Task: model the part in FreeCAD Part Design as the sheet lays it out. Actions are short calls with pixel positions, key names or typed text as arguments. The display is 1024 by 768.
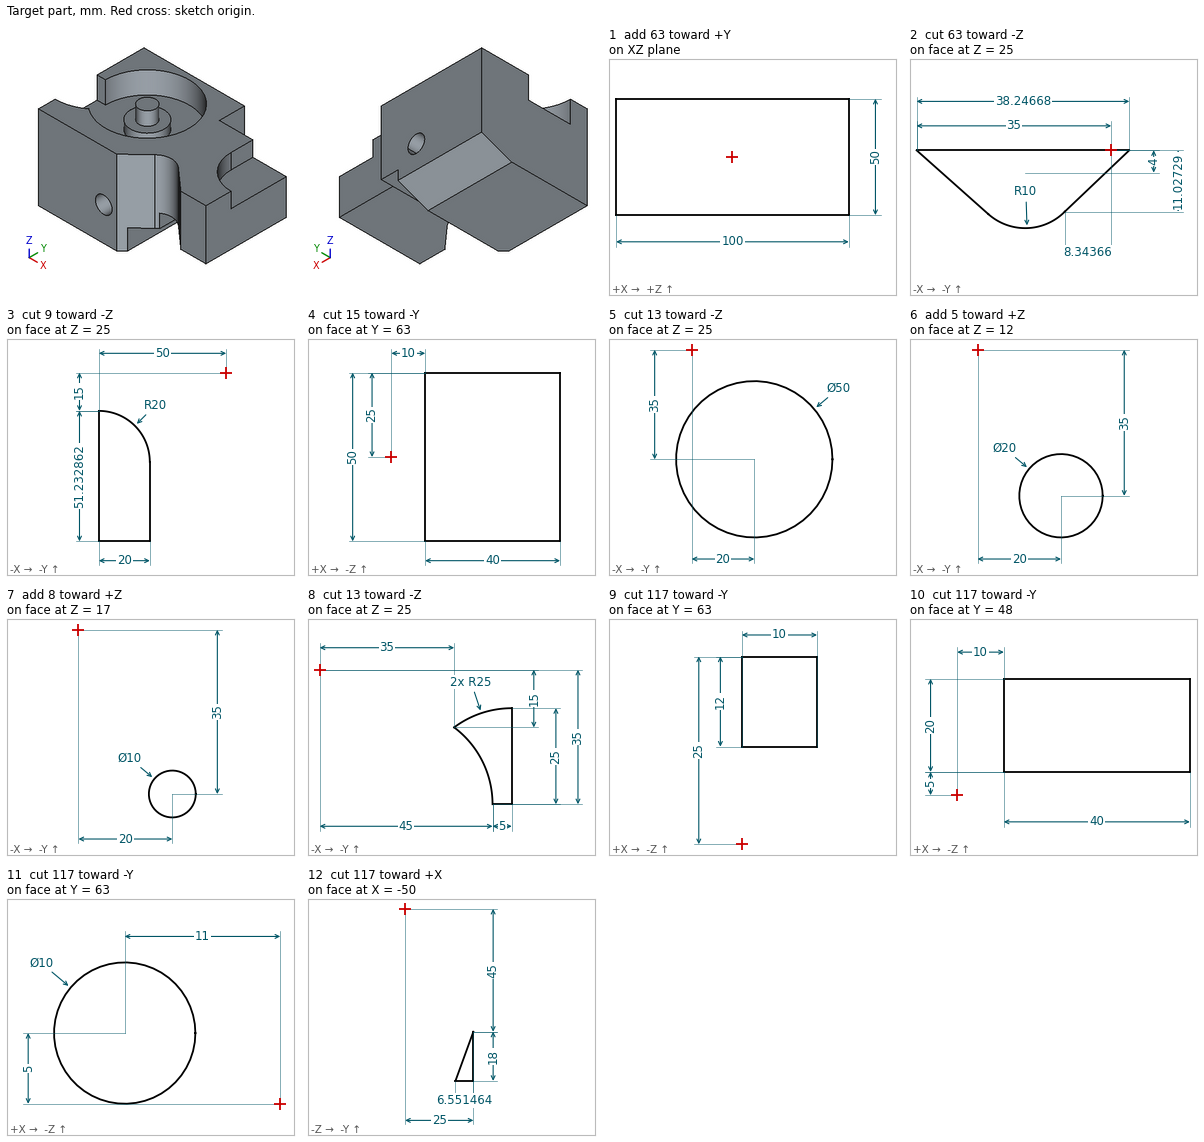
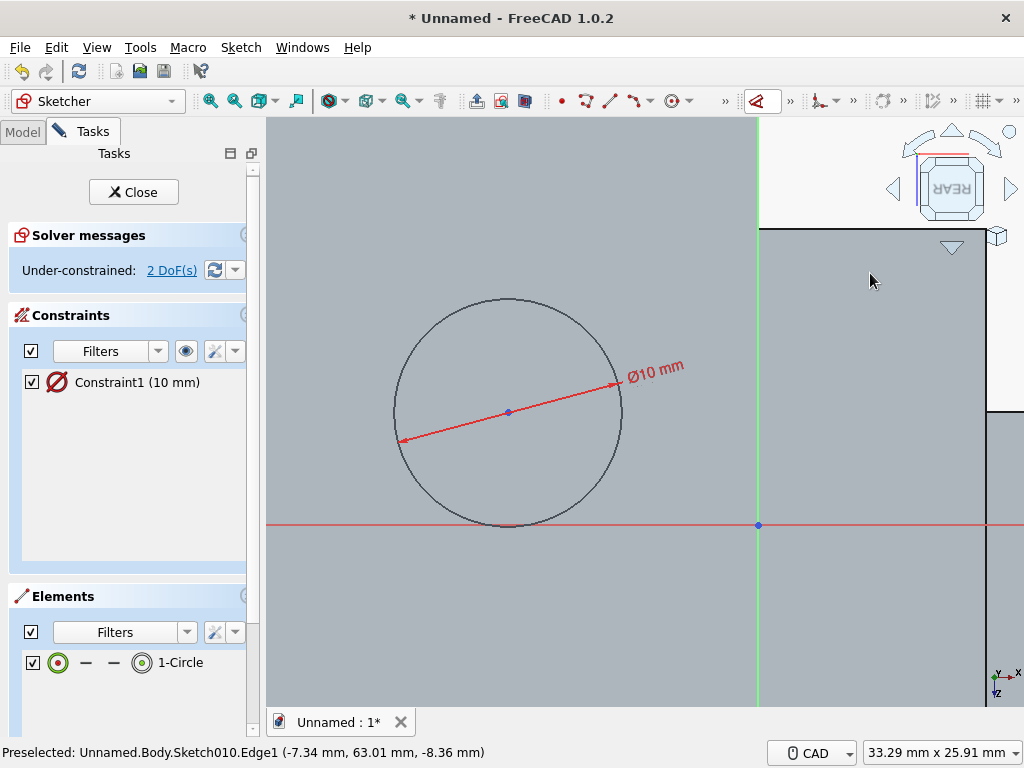
click(508, 413)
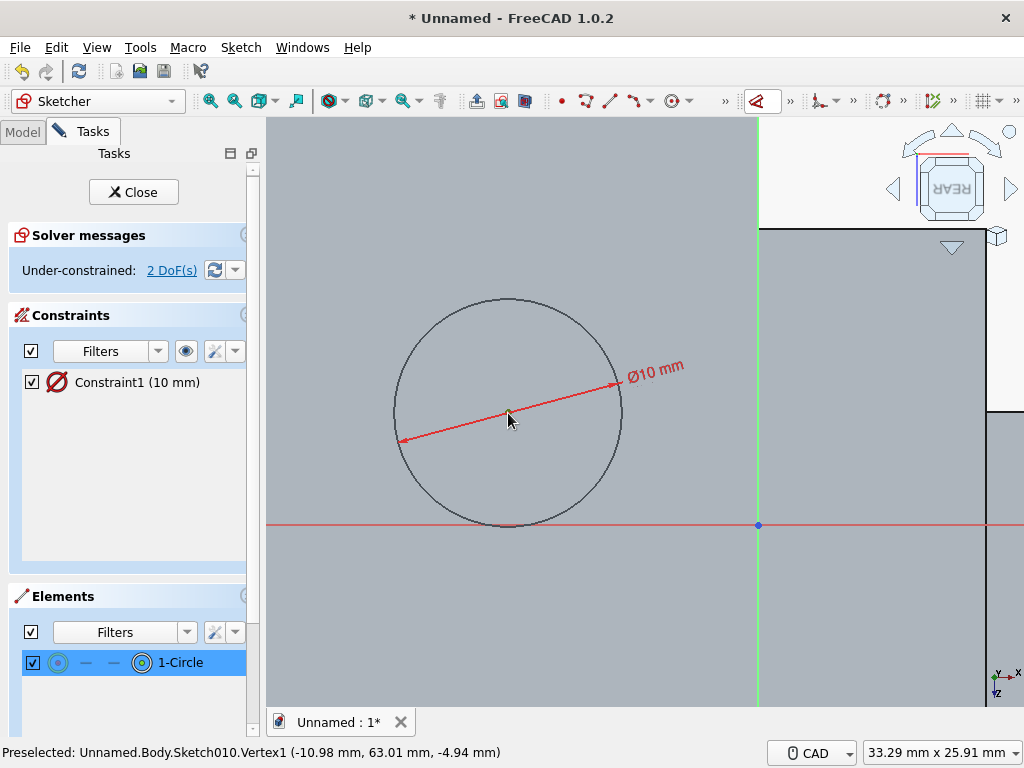
key(i)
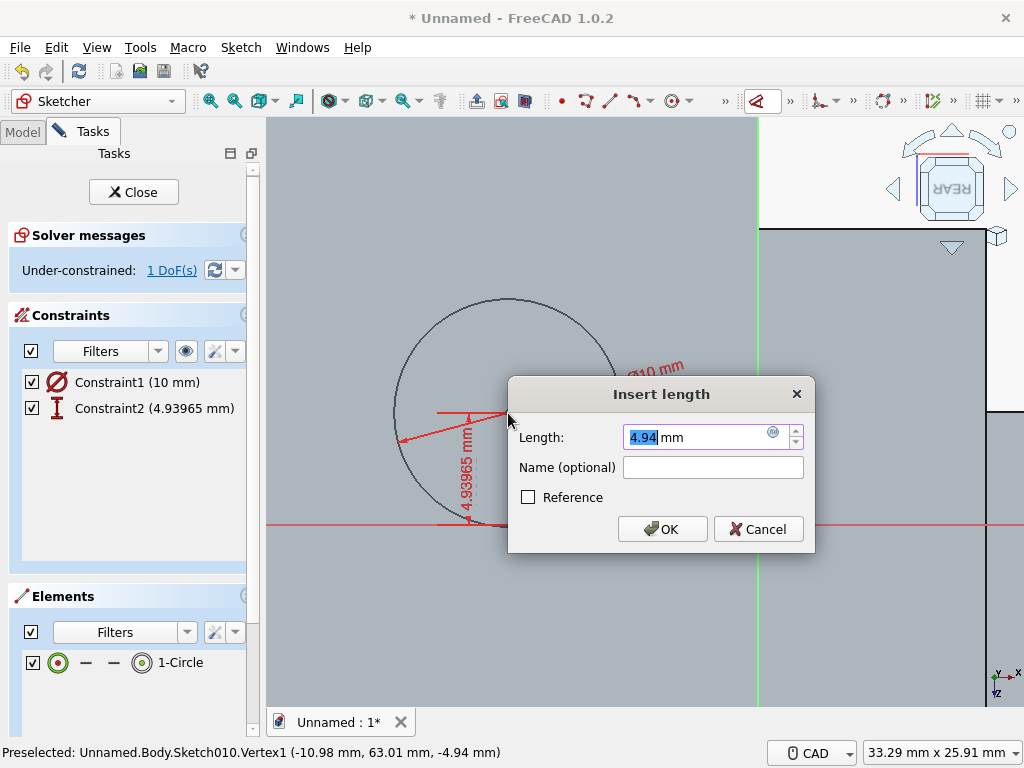
text(5)
key(Return)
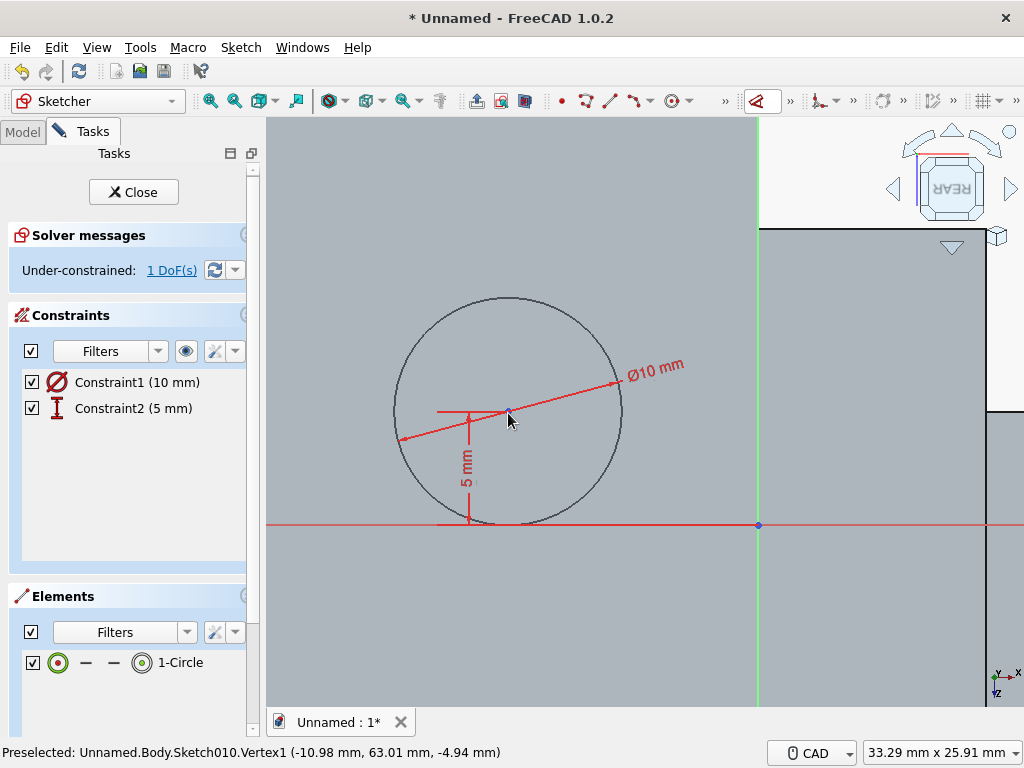
click(508, 412)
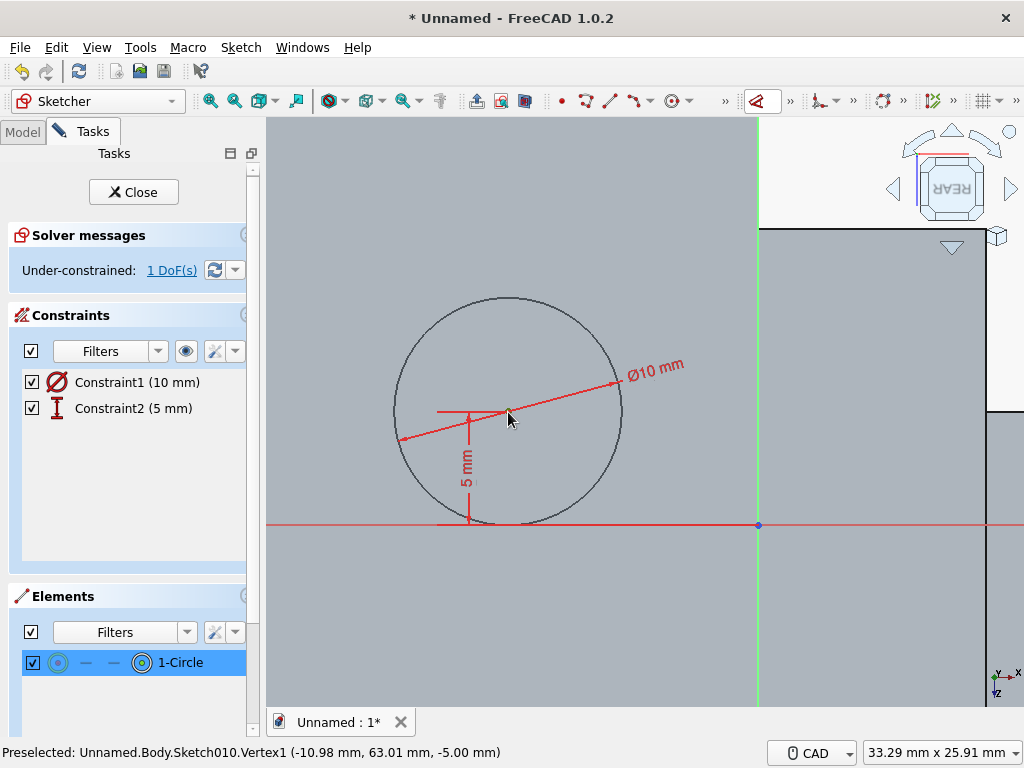
key(l)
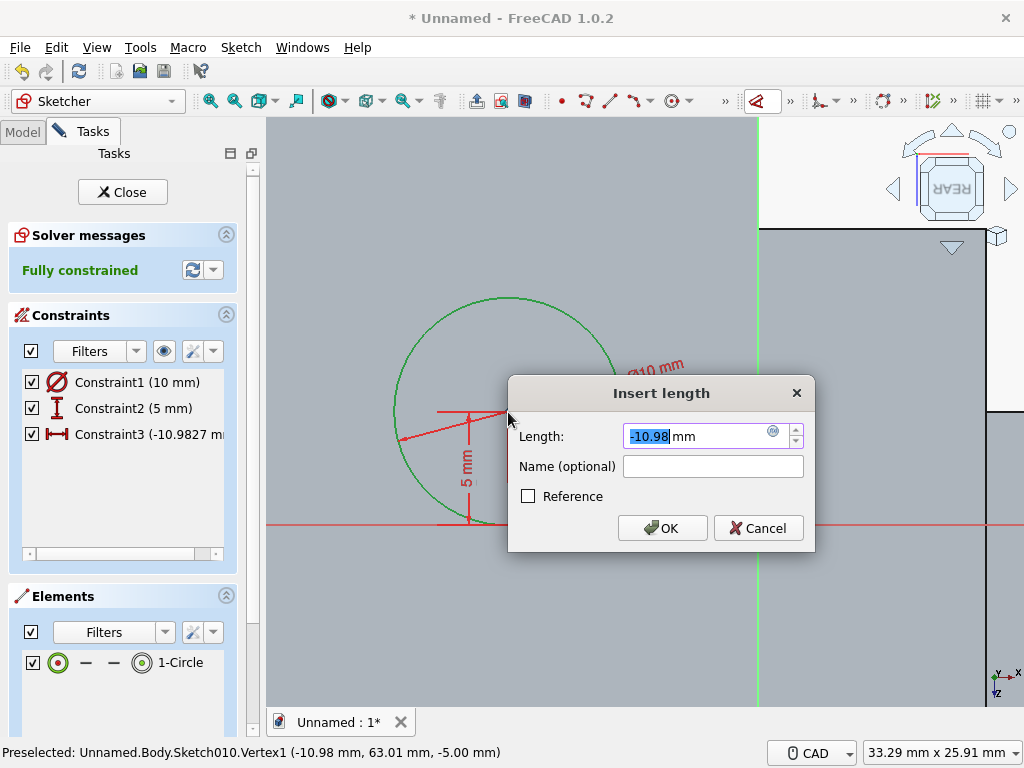
text(-11)
key(Return)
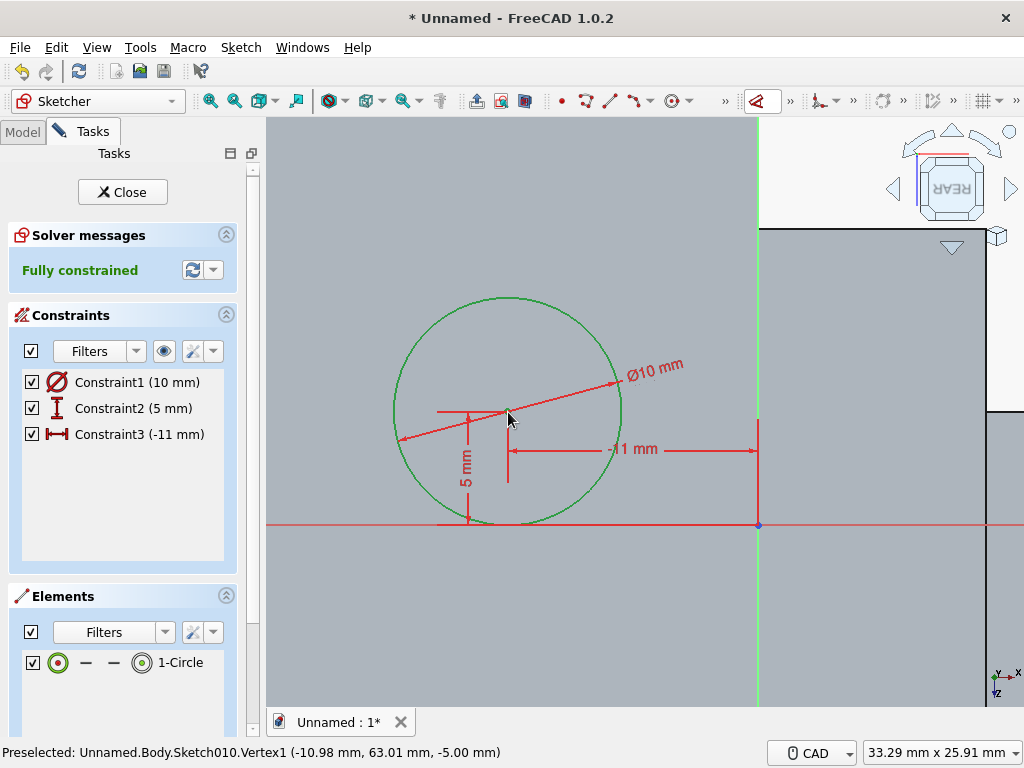
click(123, 192)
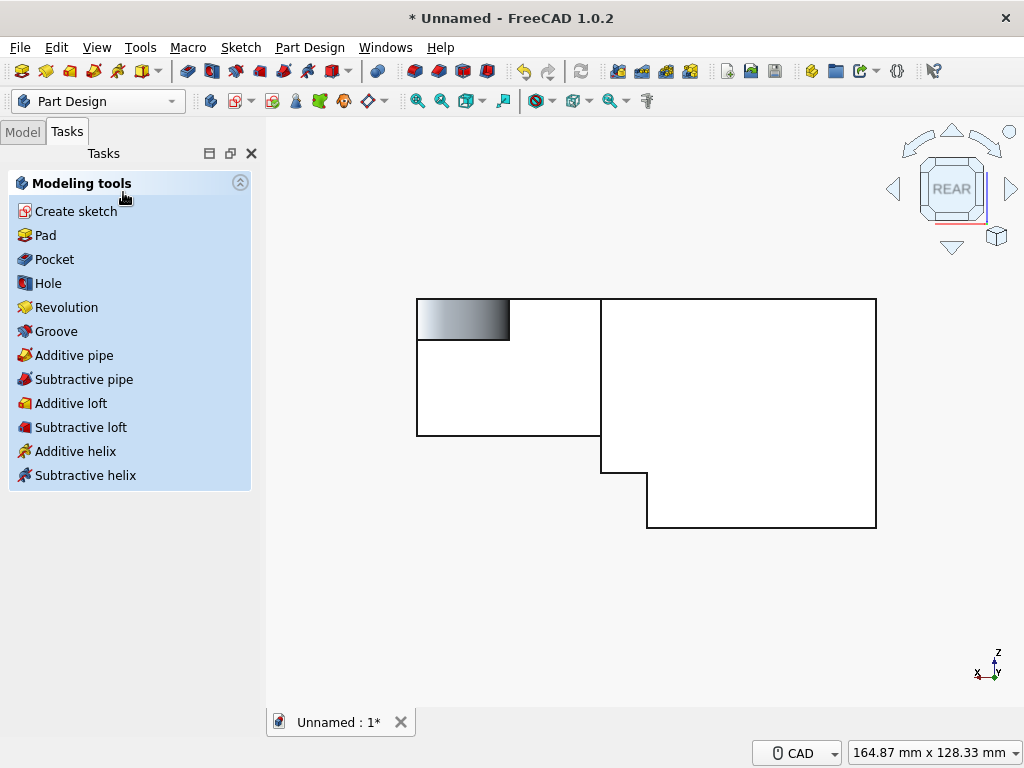
click(188, 72)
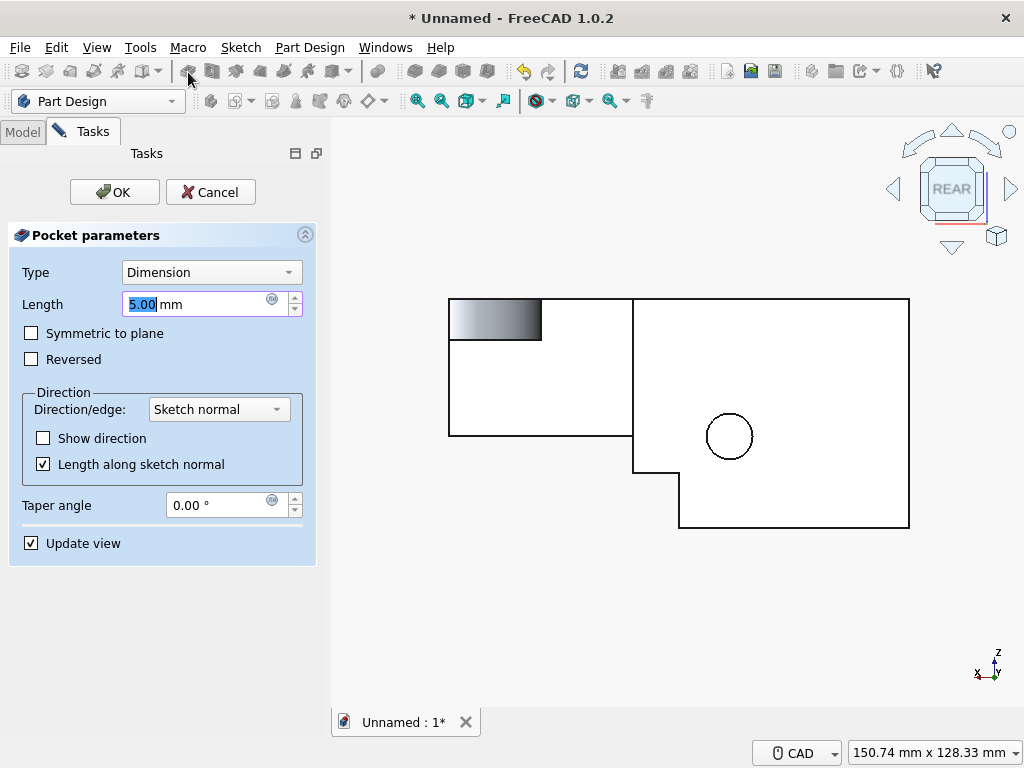
text(117)
key(Tab)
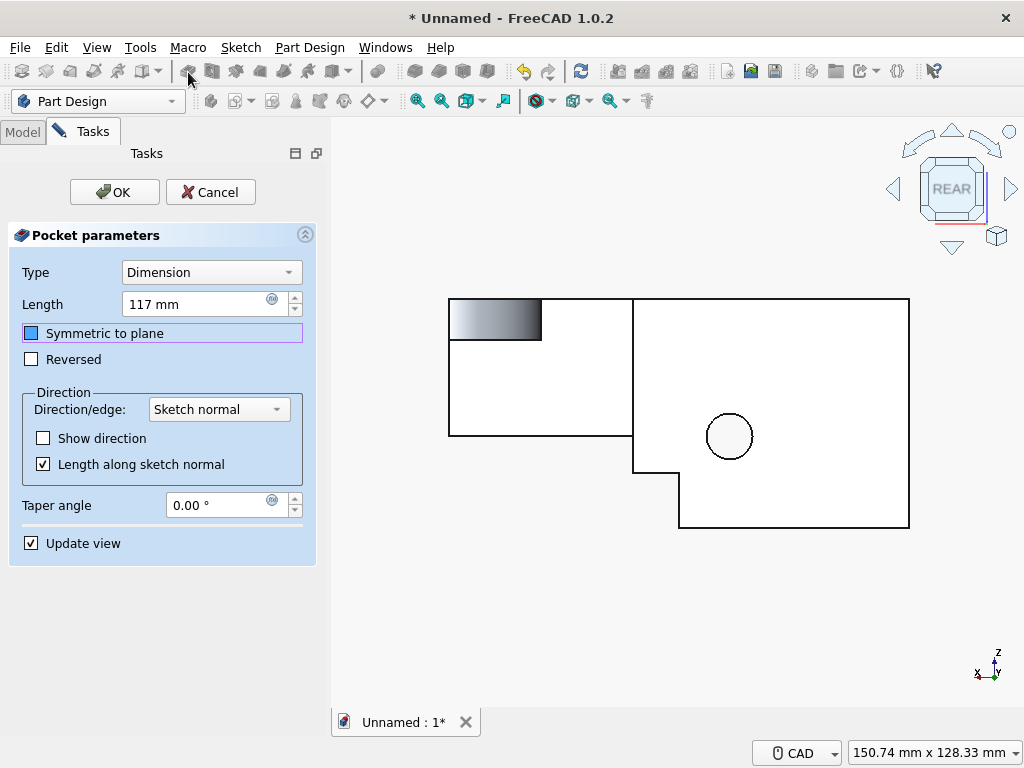
click(115, 192)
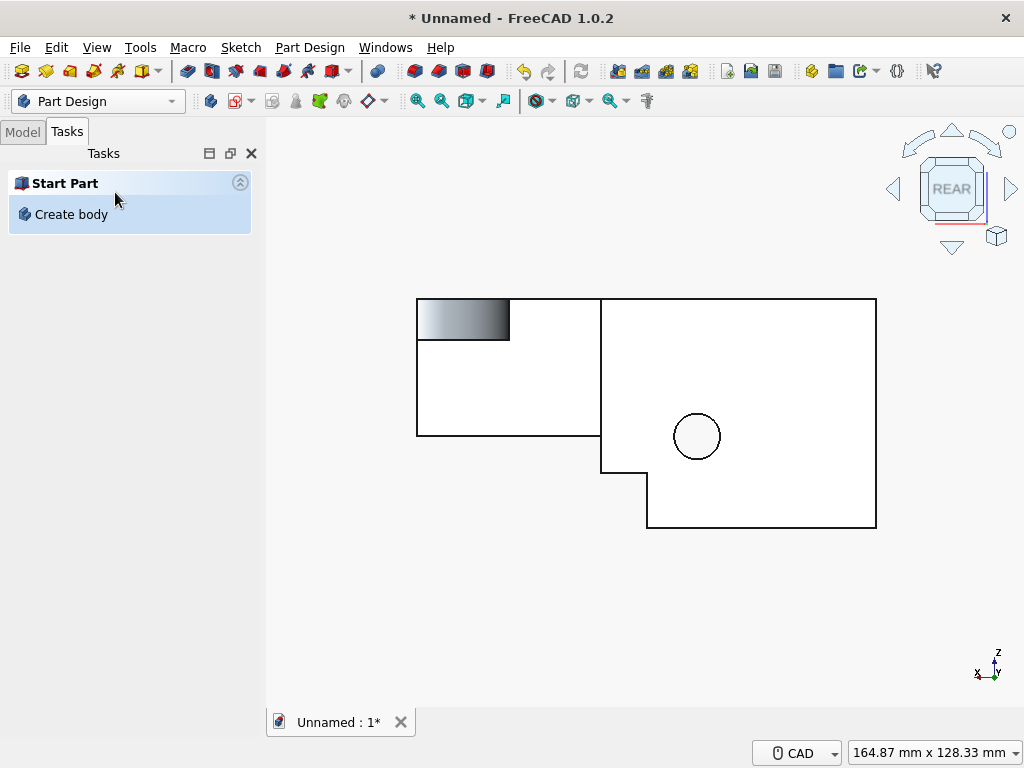
key(6)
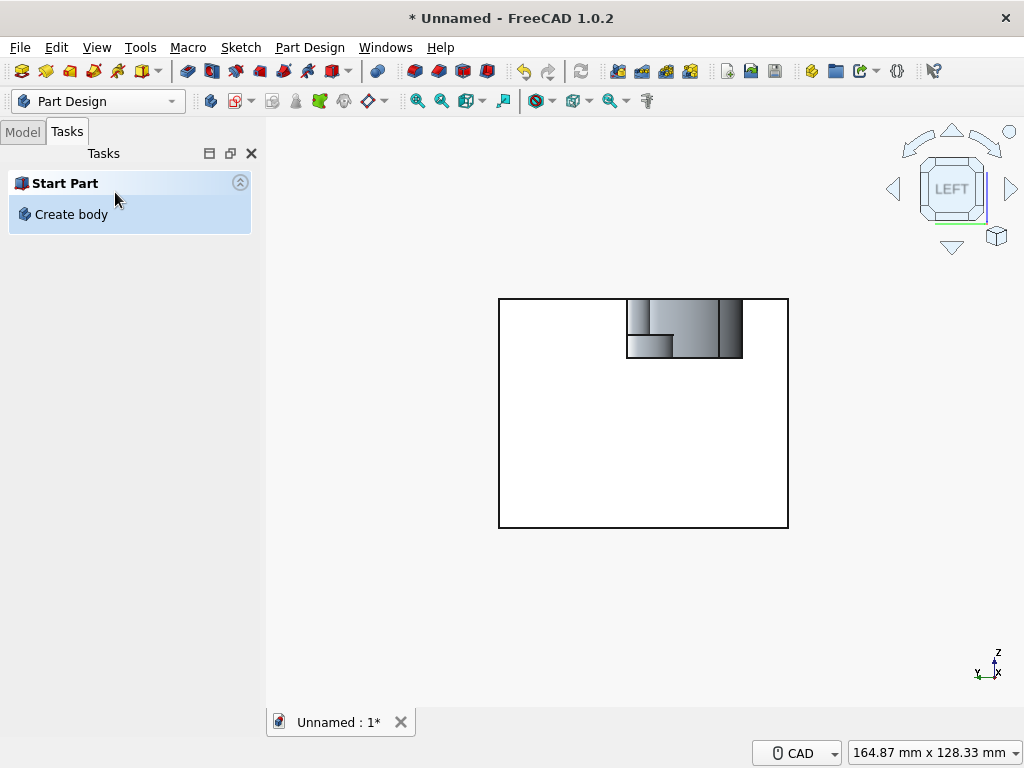
click(418, 102)